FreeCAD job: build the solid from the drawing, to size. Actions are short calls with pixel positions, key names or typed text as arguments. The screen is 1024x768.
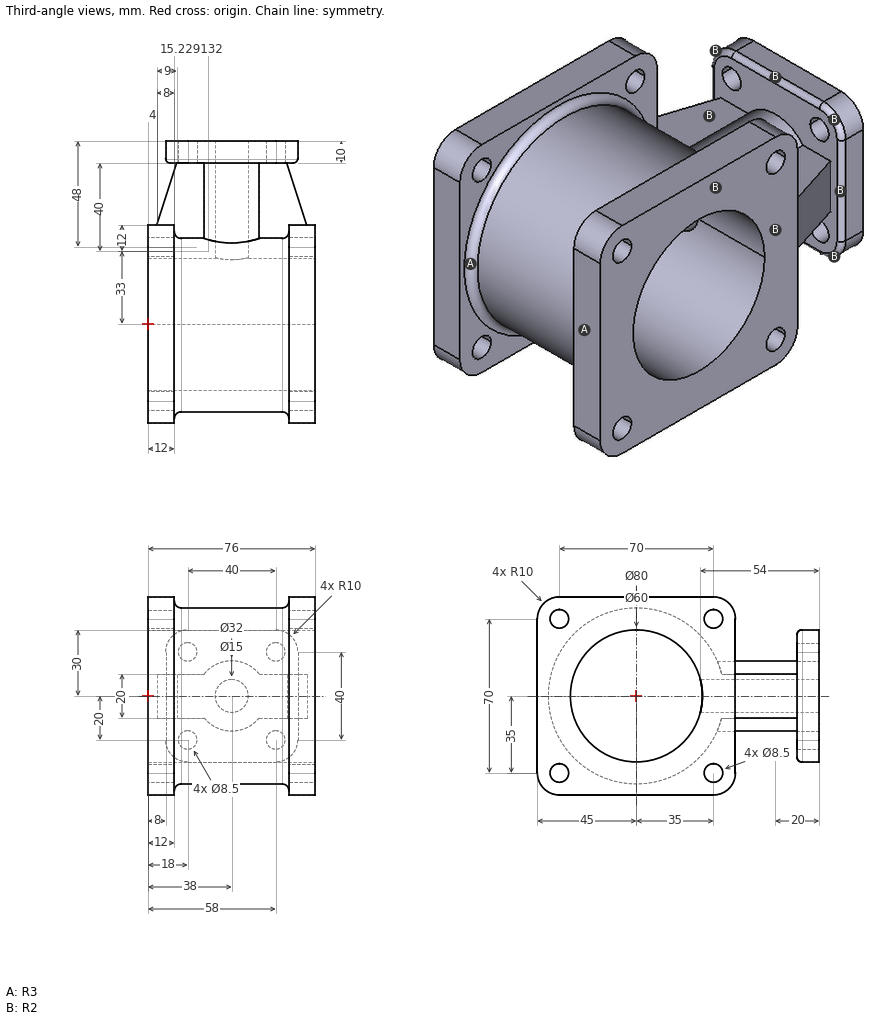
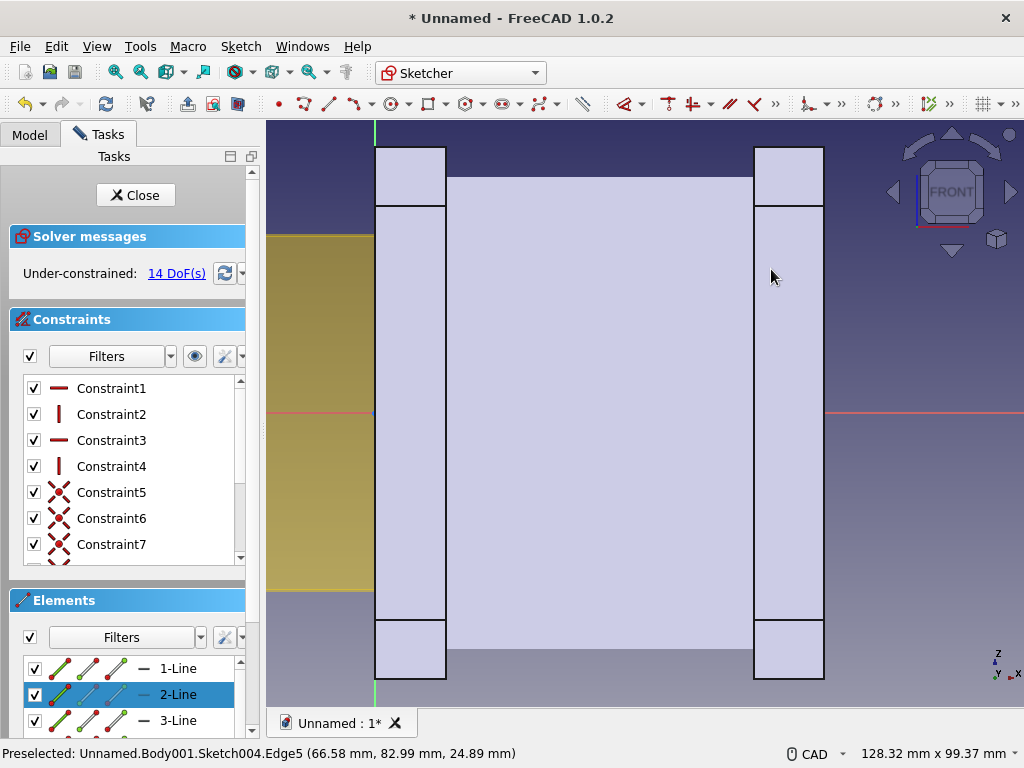
key(t)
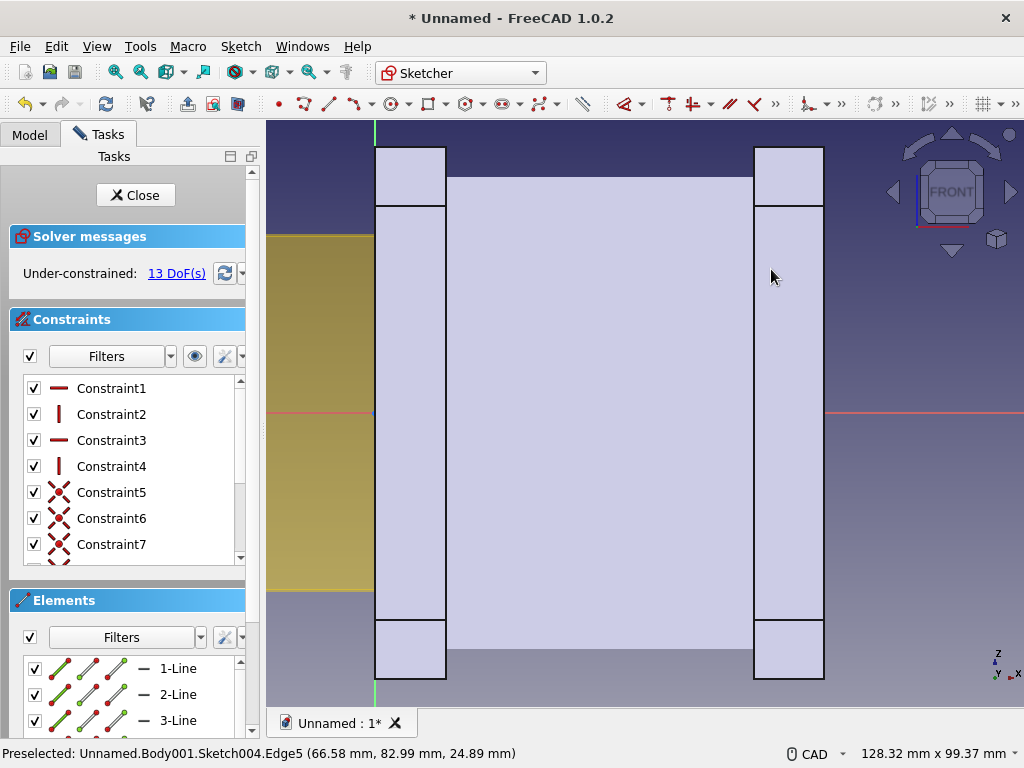
click(777, 367)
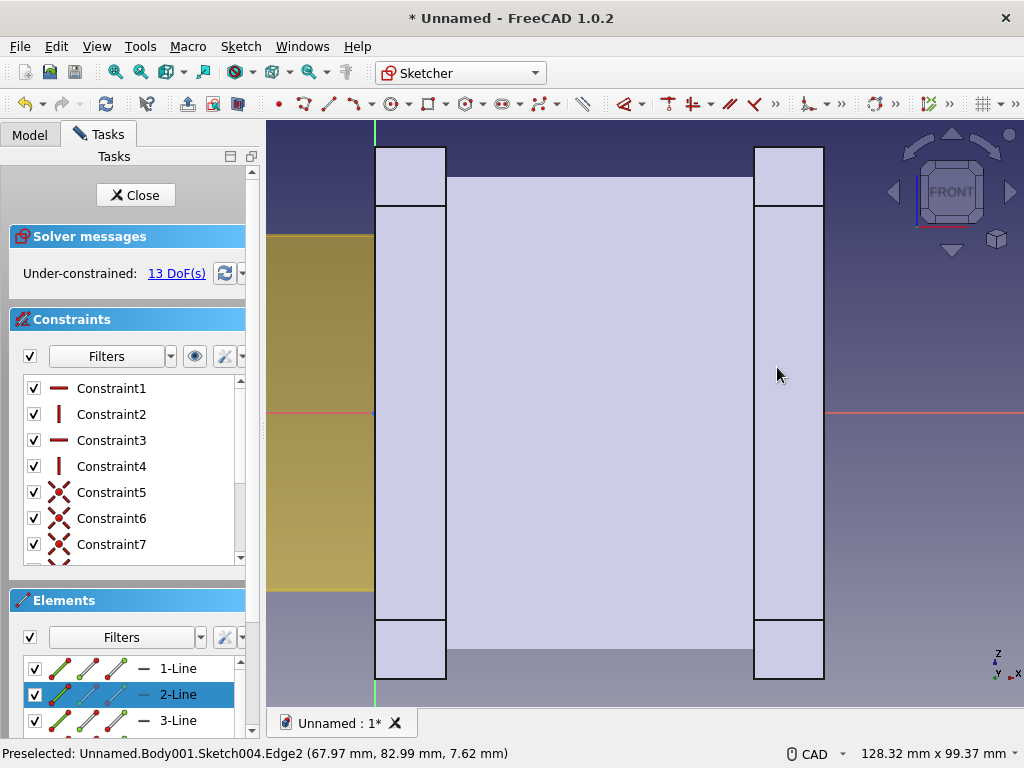
click(745, 585)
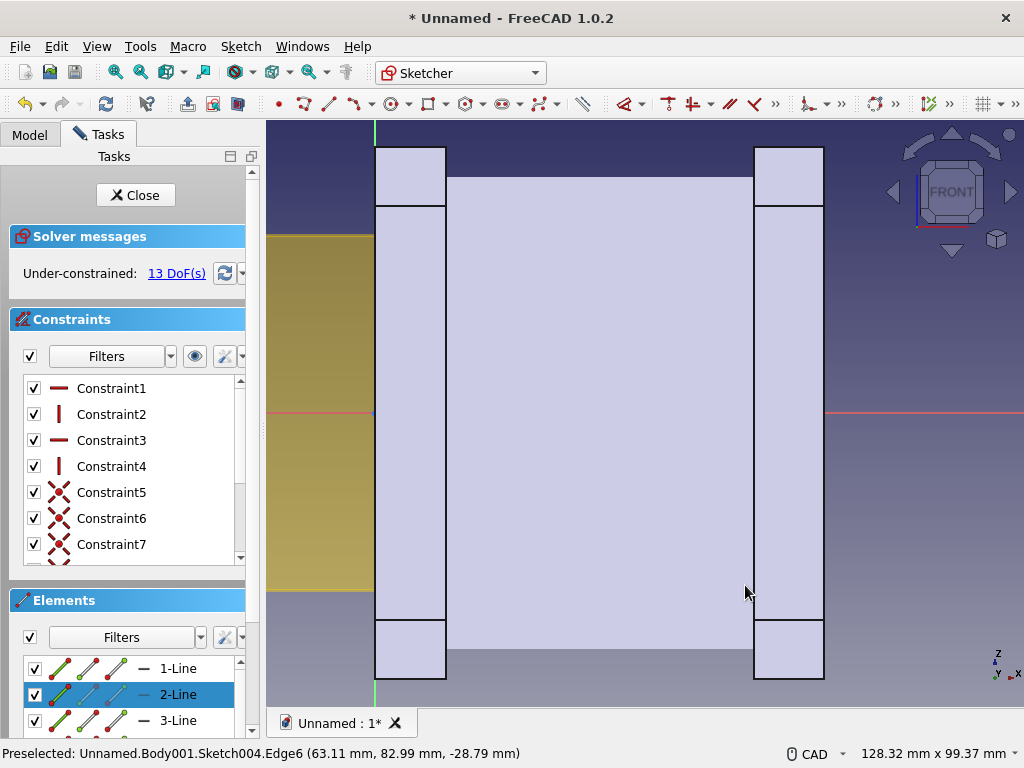
key(t)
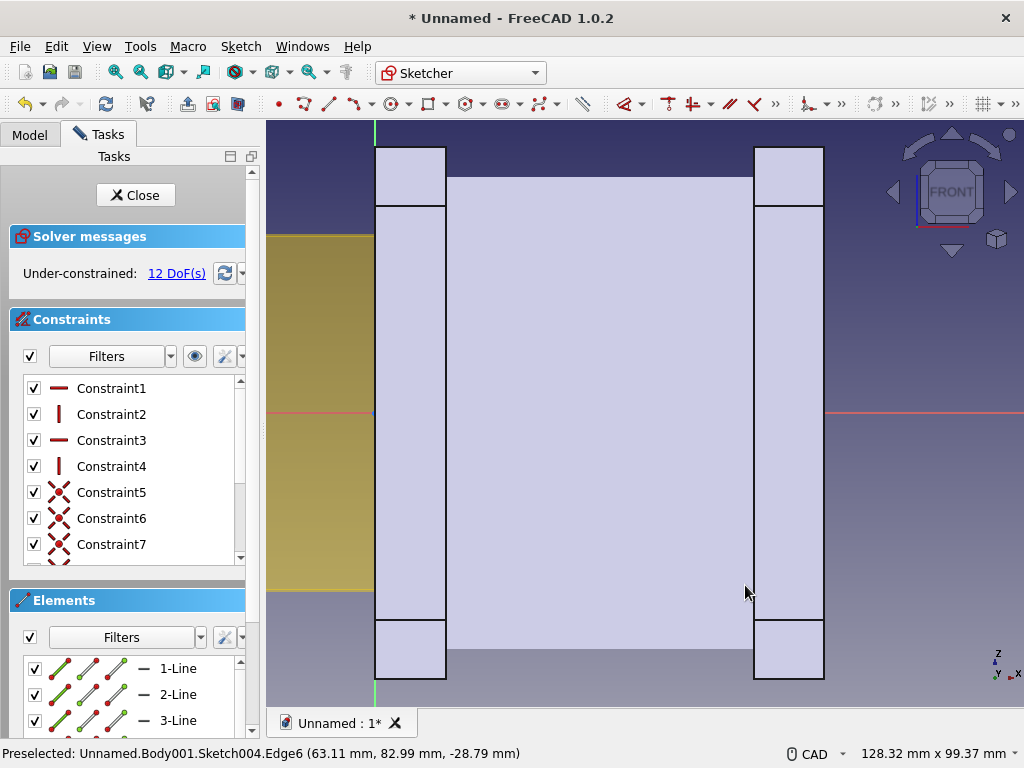
click(647, 591)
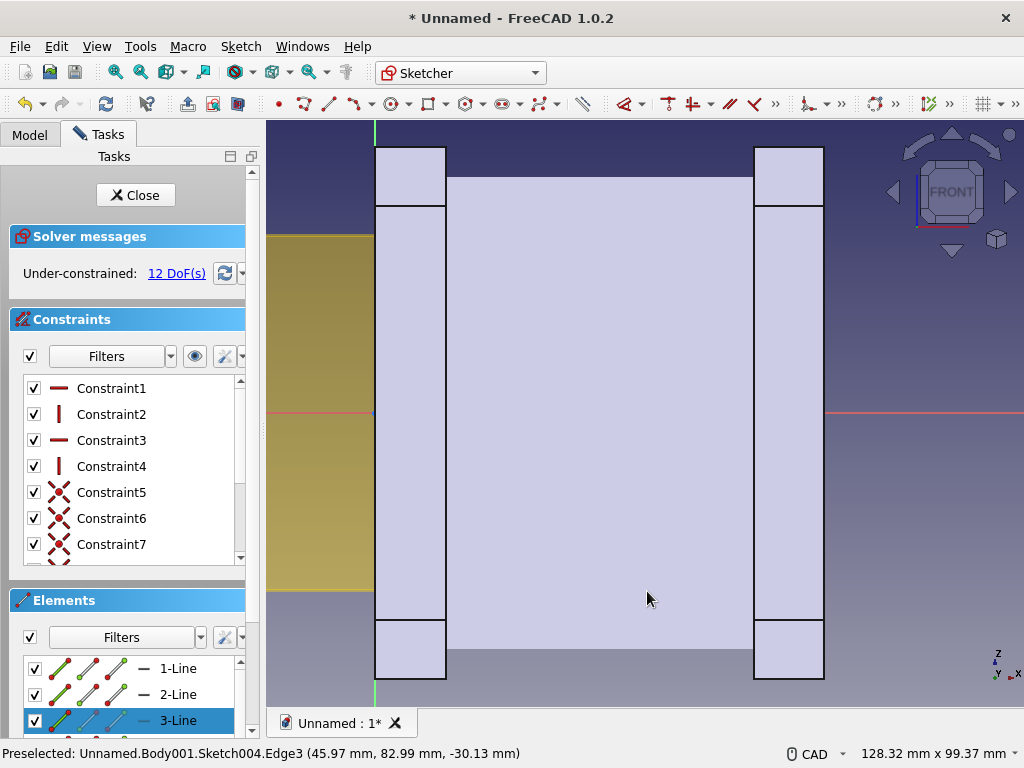
click(745, 585)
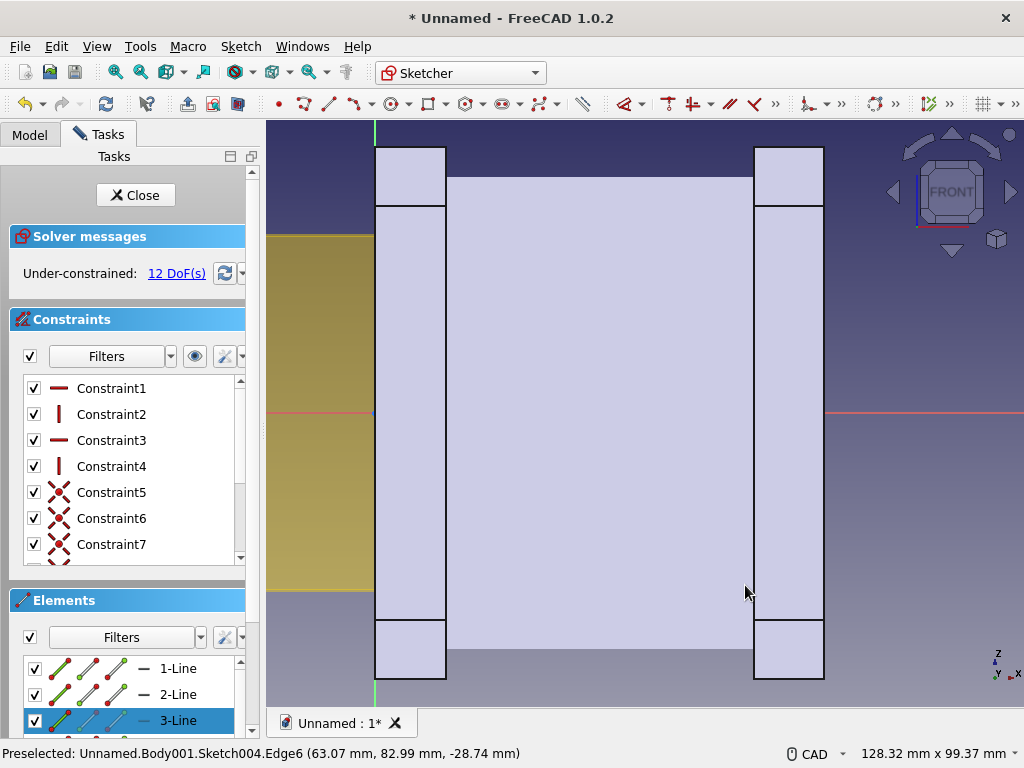
key(t)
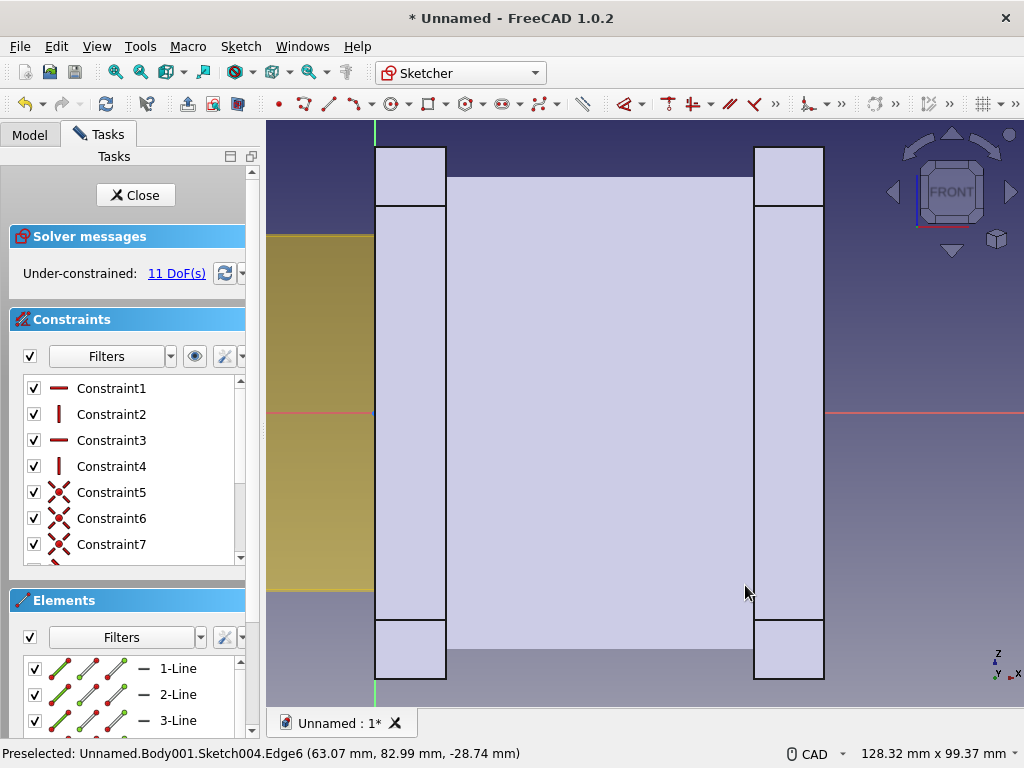
click(647, 591)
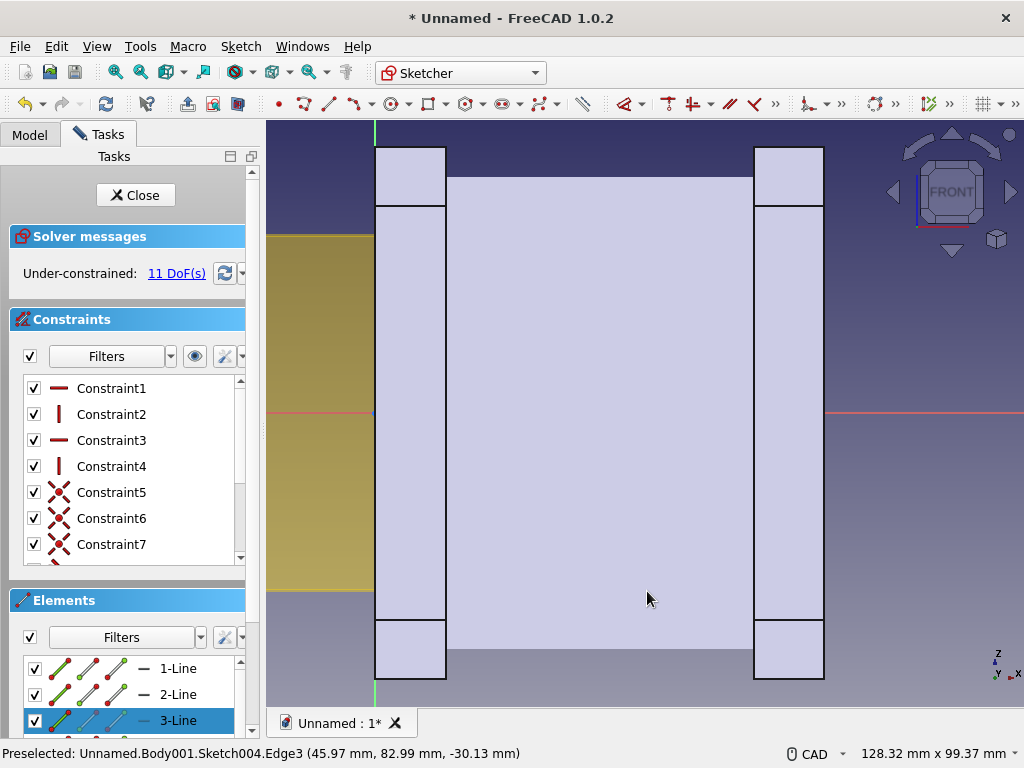
click(429, 559)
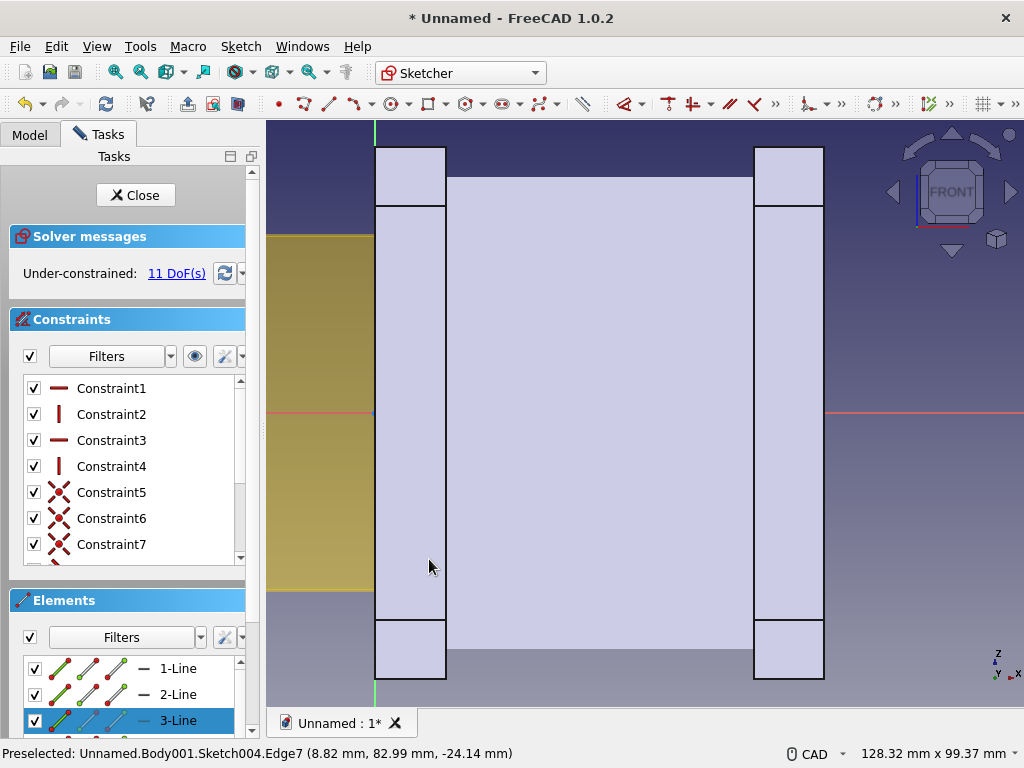
key(t)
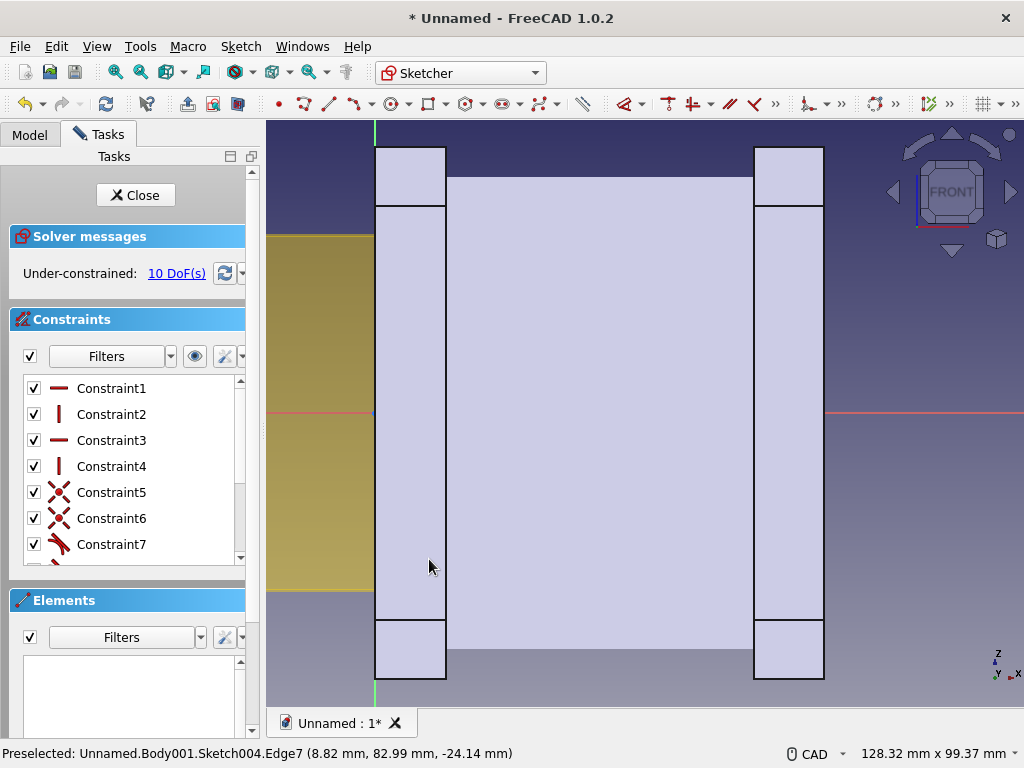
click(423, 461)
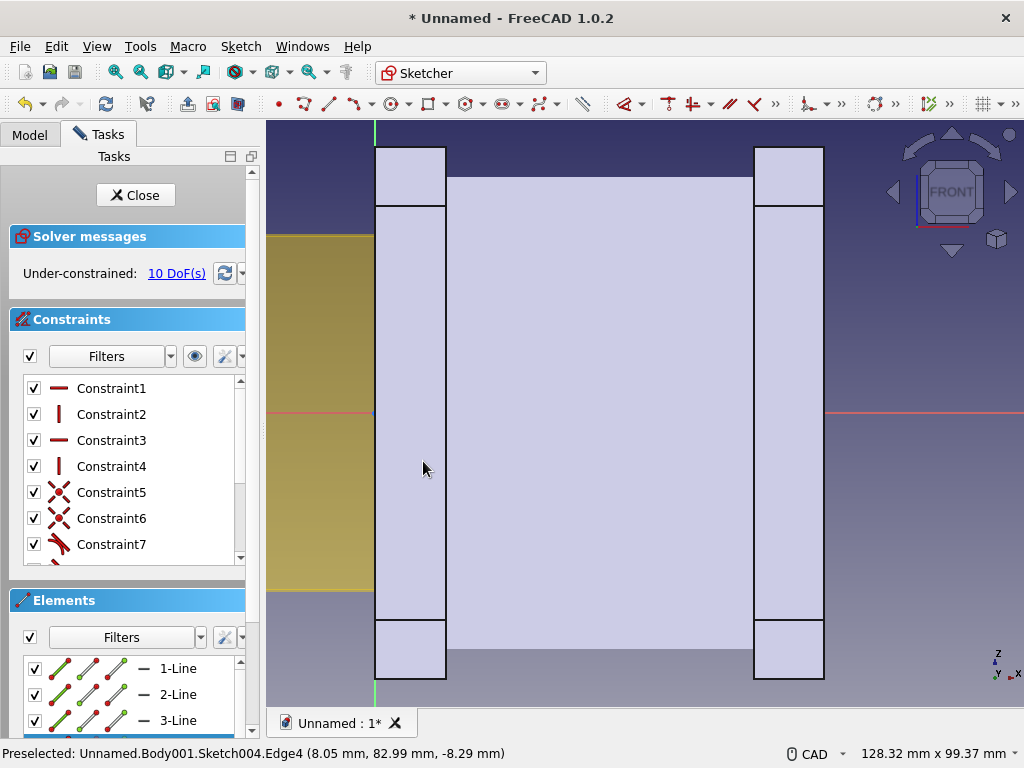
click(429, 559)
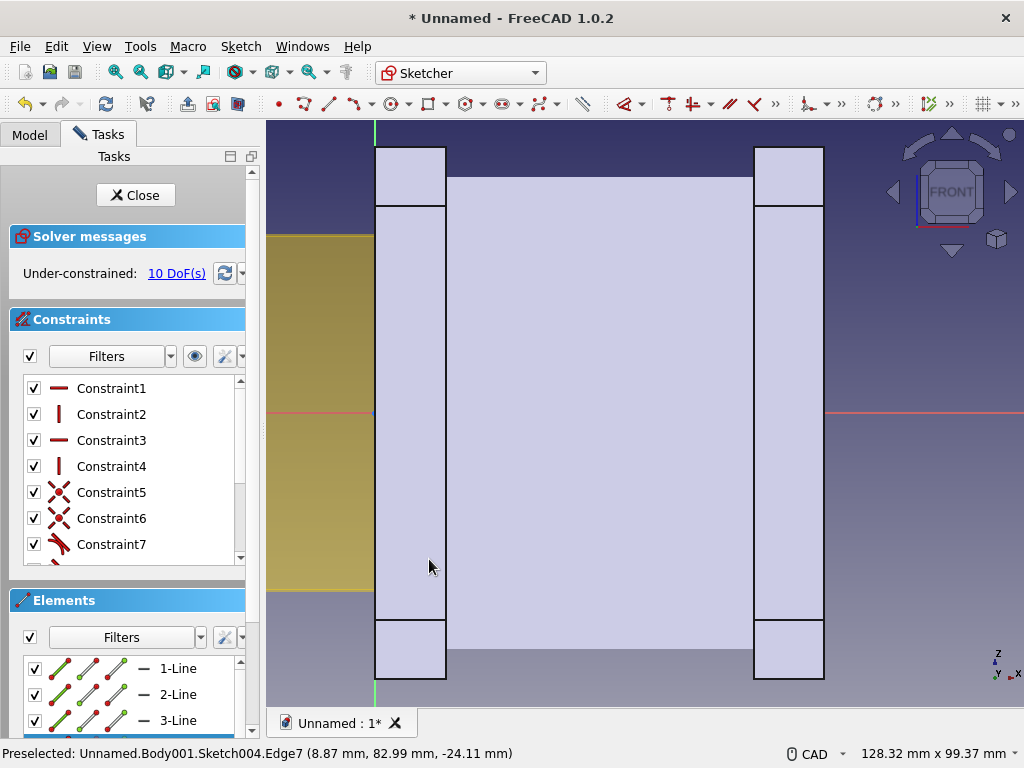
key(t)